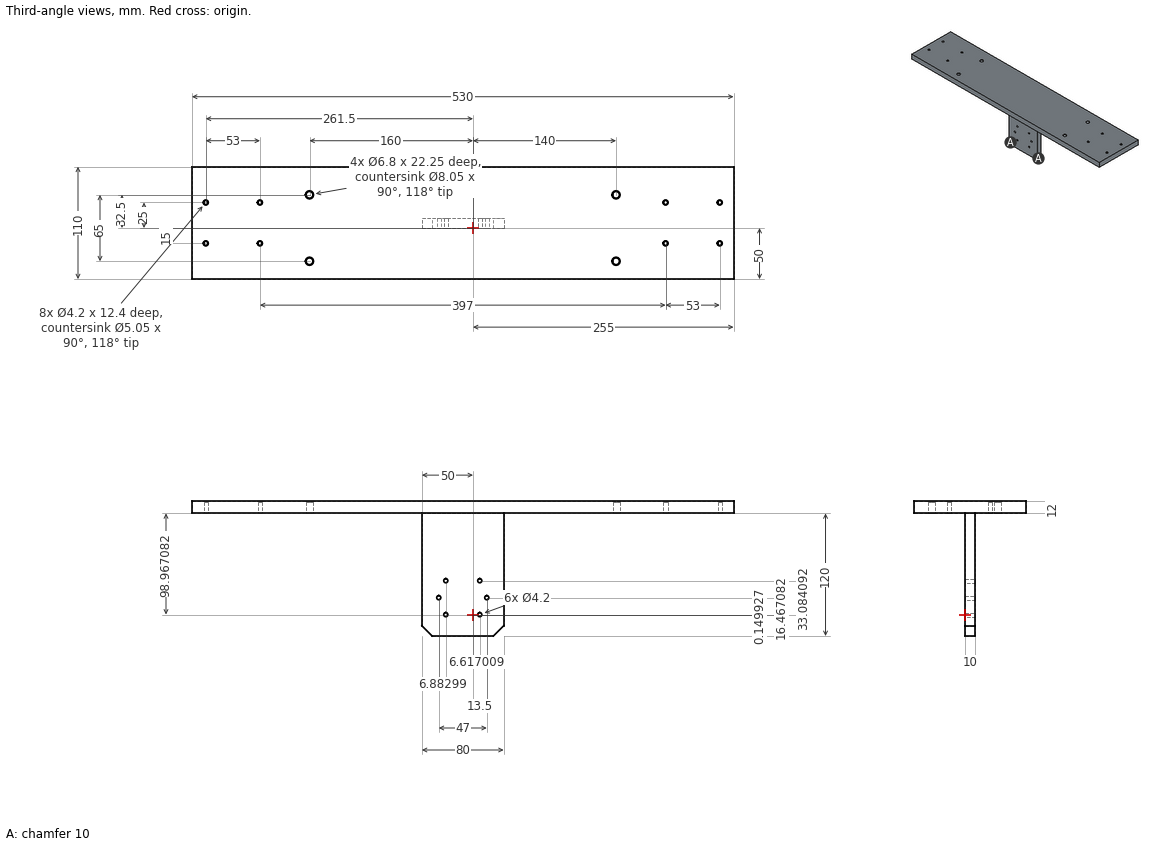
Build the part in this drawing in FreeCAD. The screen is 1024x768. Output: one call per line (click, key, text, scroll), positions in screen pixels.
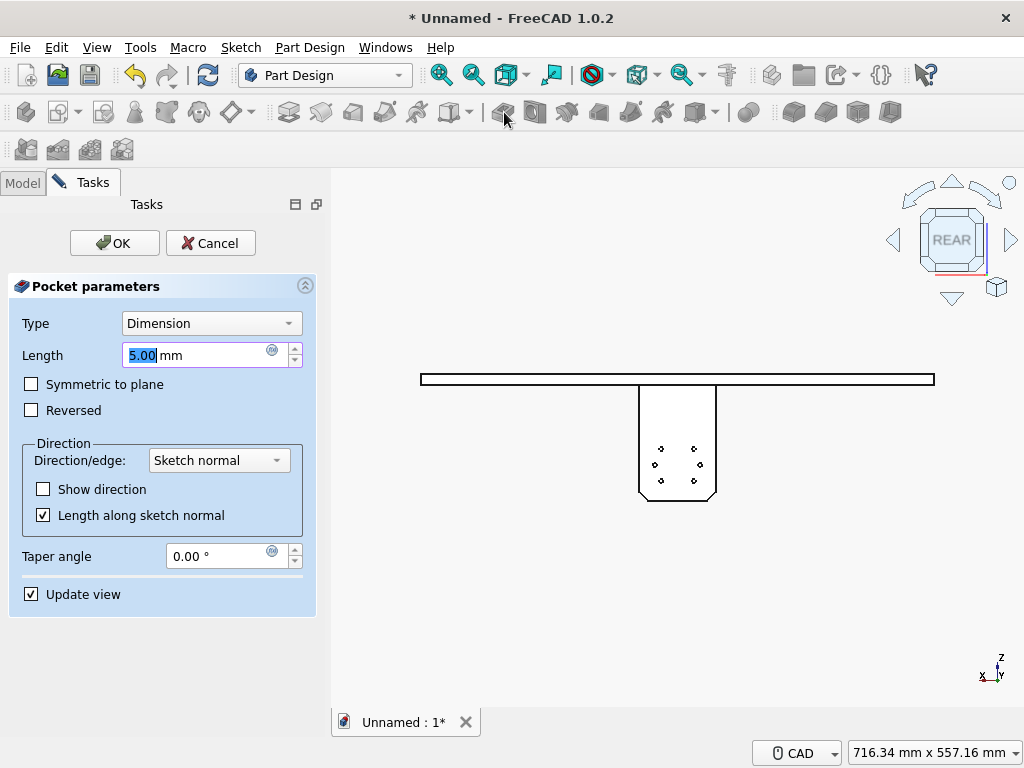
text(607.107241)
key(Tab)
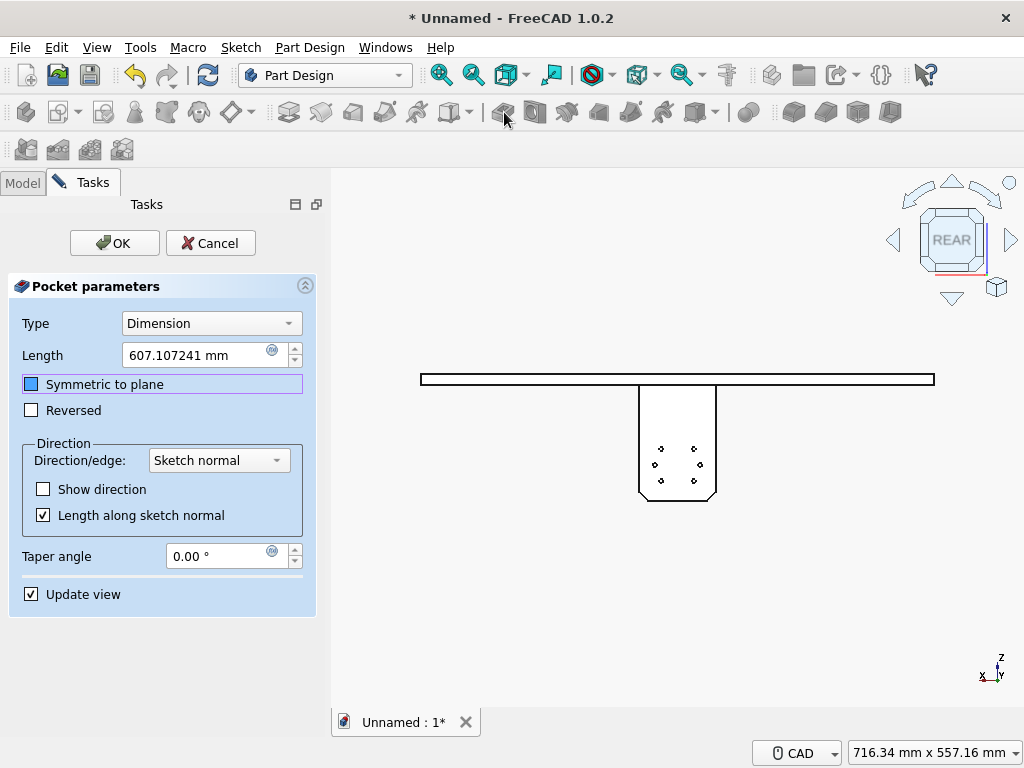
click(30, 384)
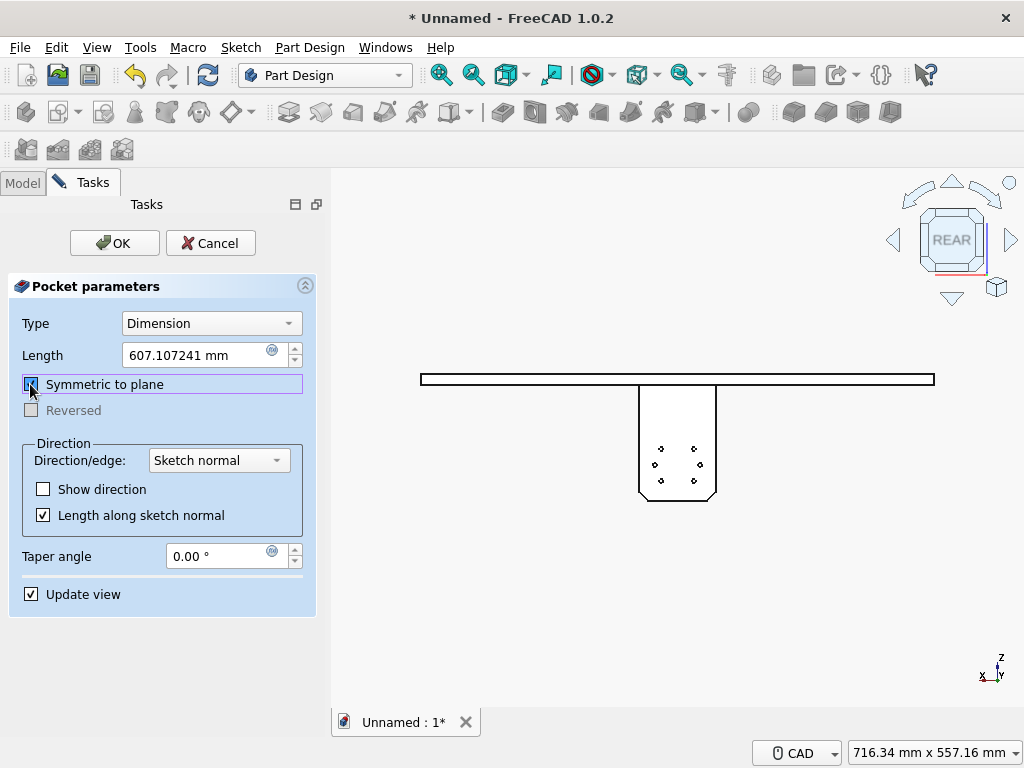
click(115, 243)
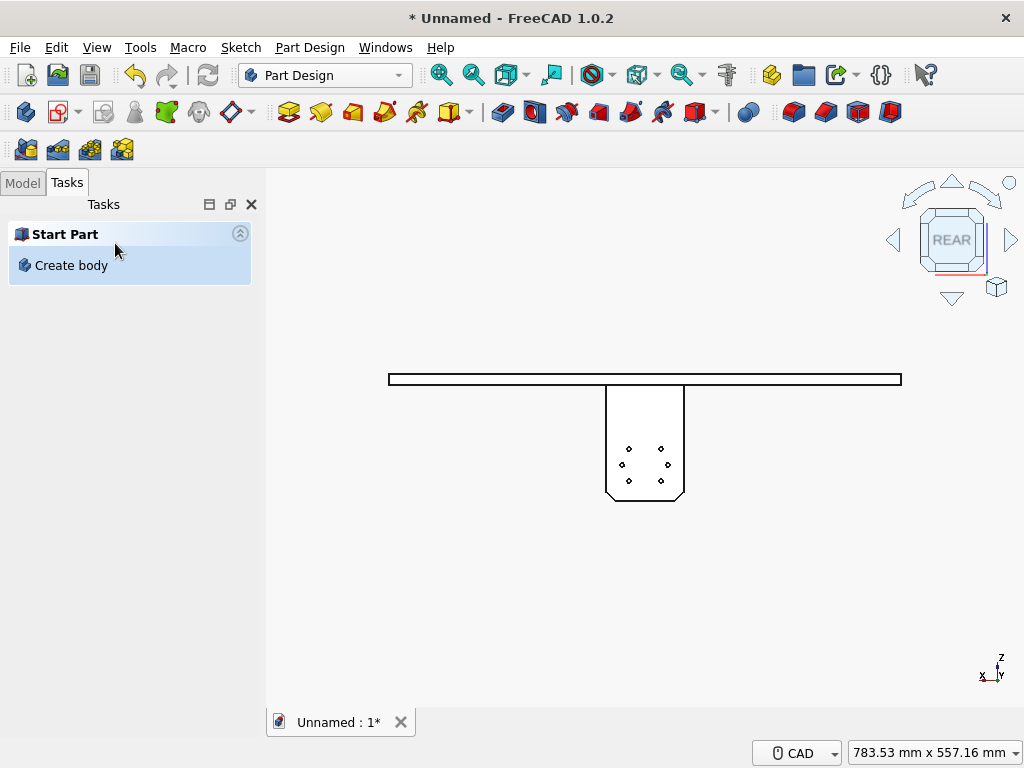
key(0)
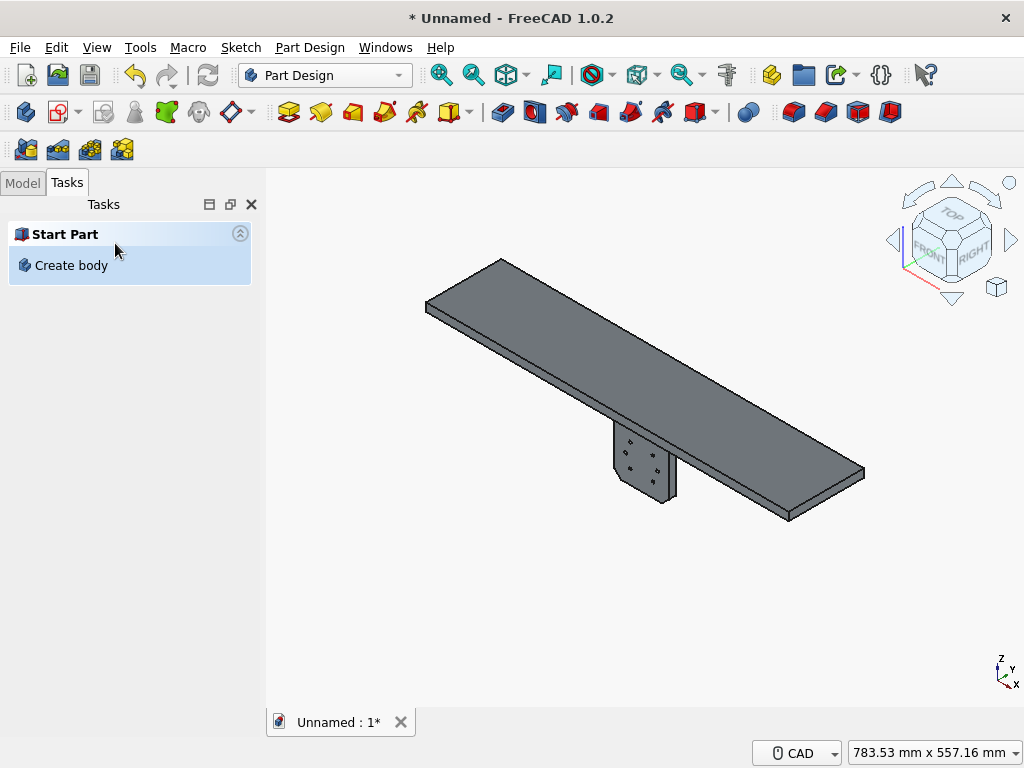
click(749, 444)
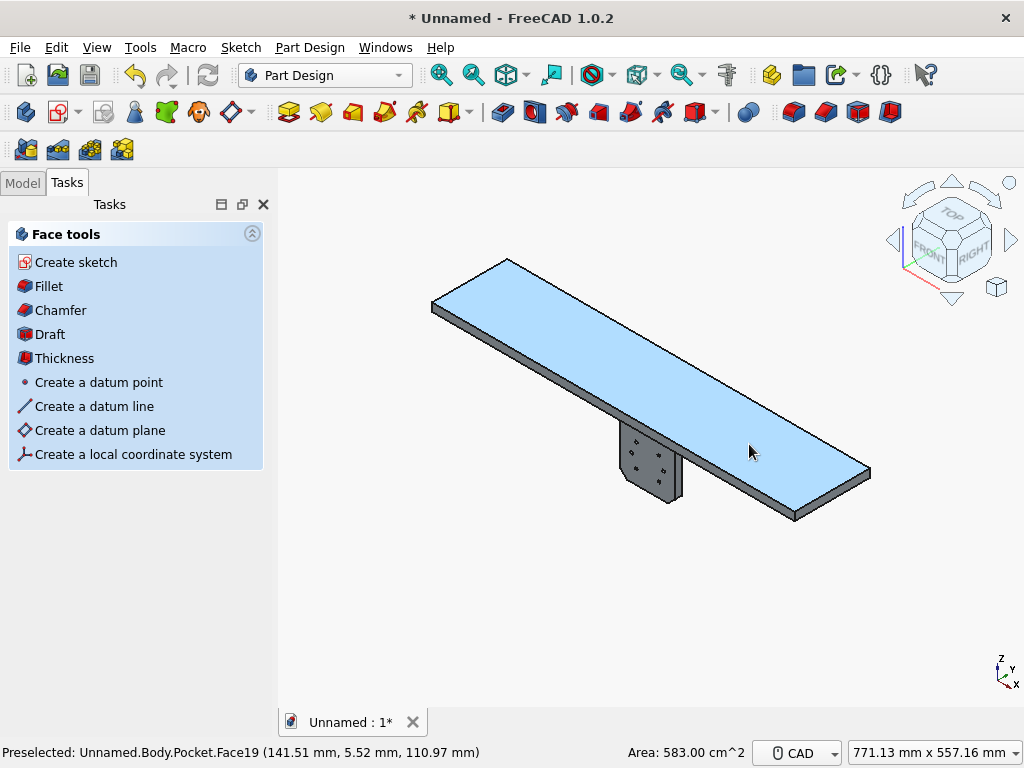
click(58, 112)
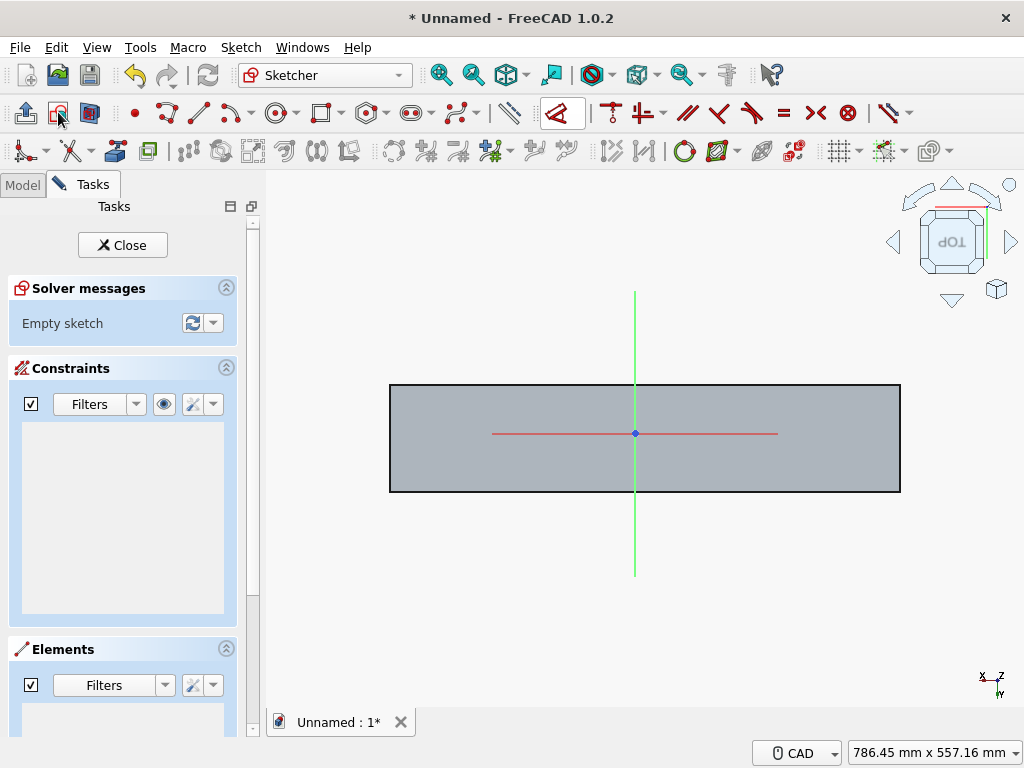
scroll(294, 439, down, 1)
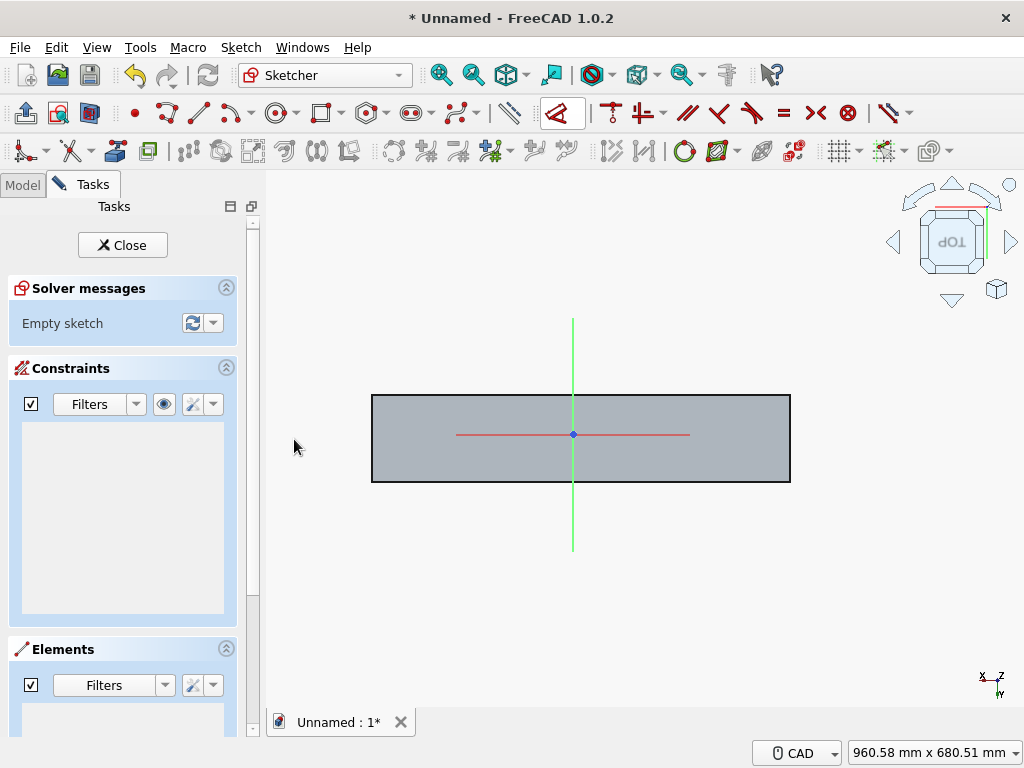
click(276, 114)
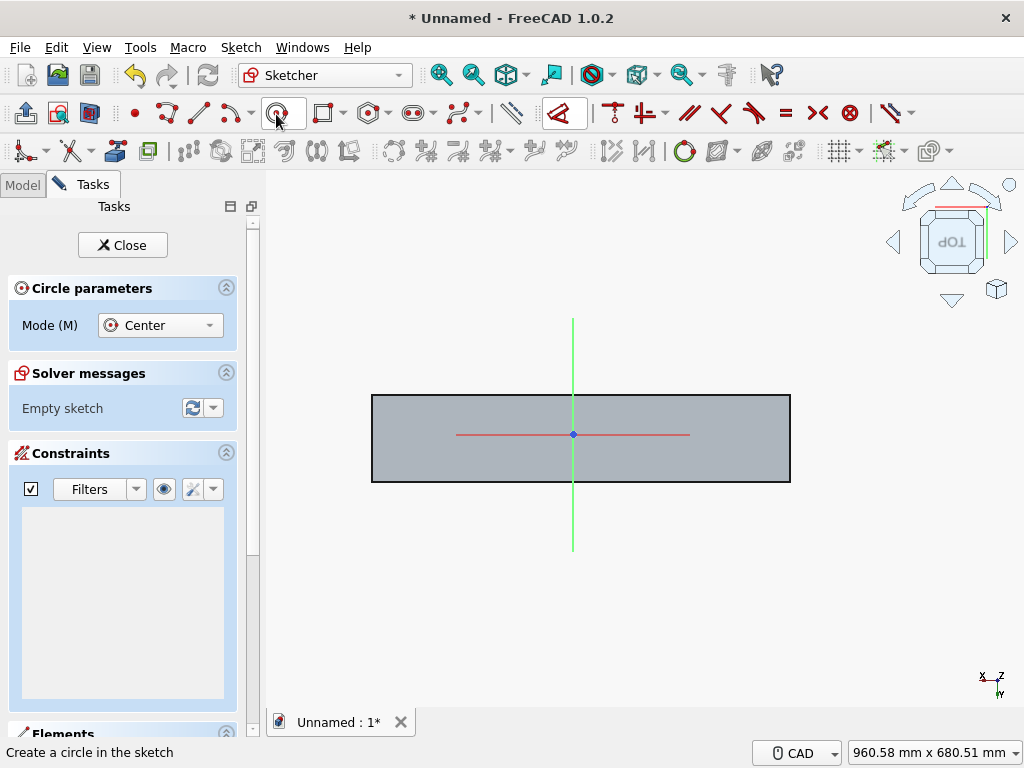
scroll(780, 454, up, 14)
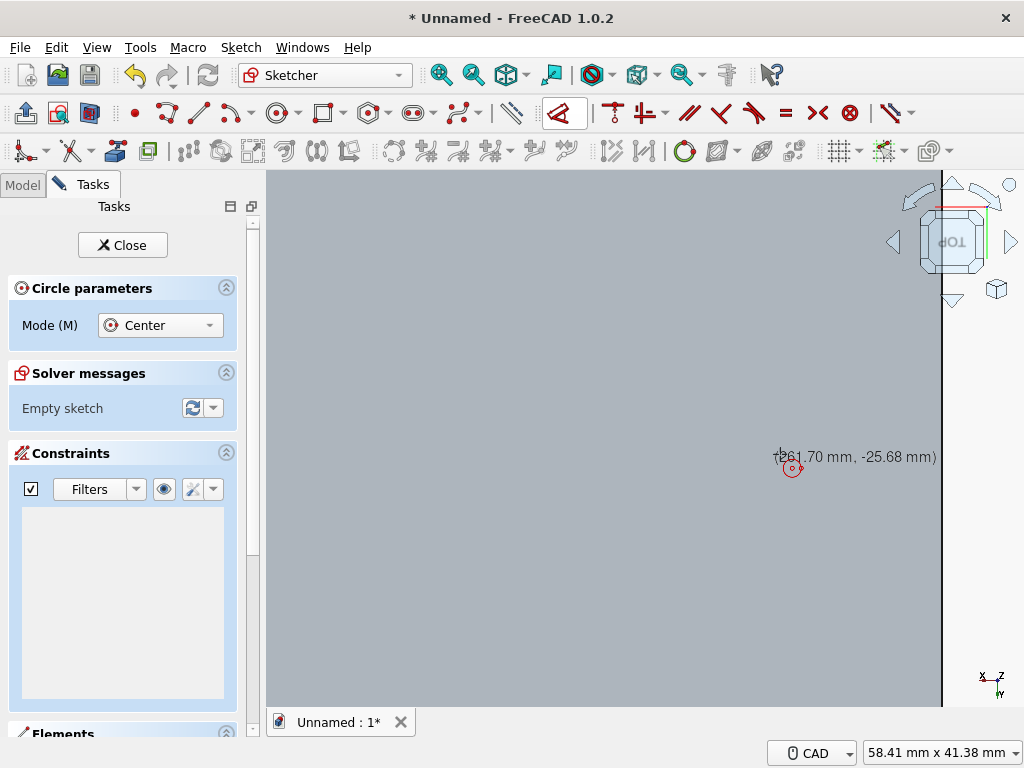
scroll(775, 454, down, 14)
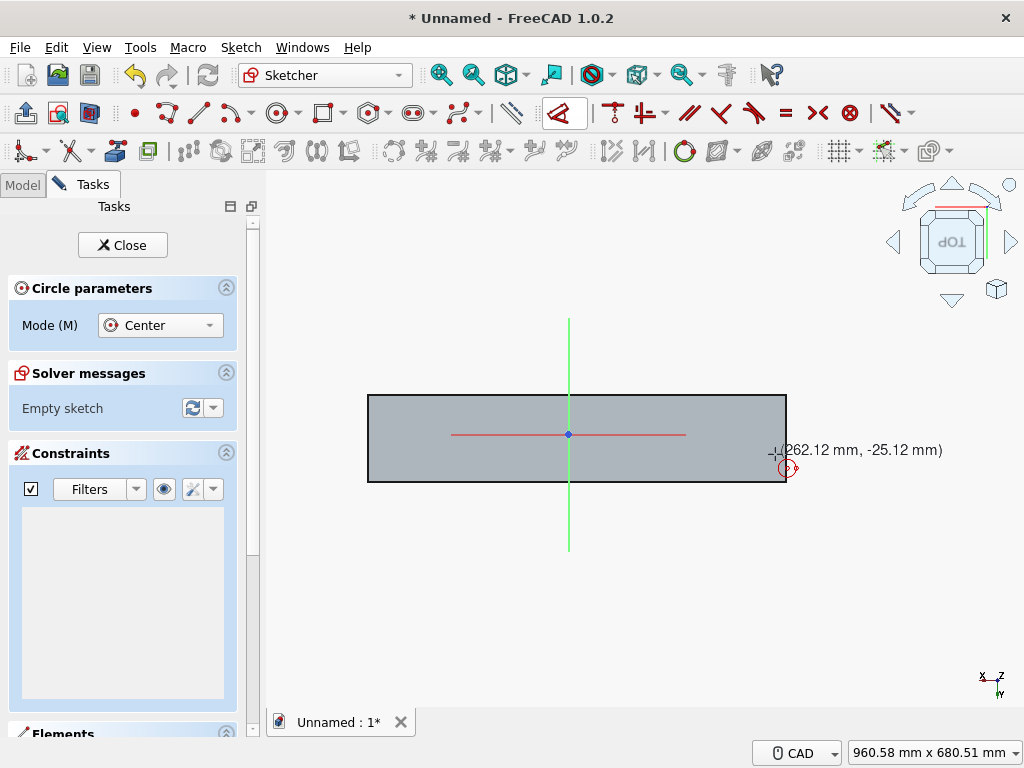
click(775, 454)
move(776, 453)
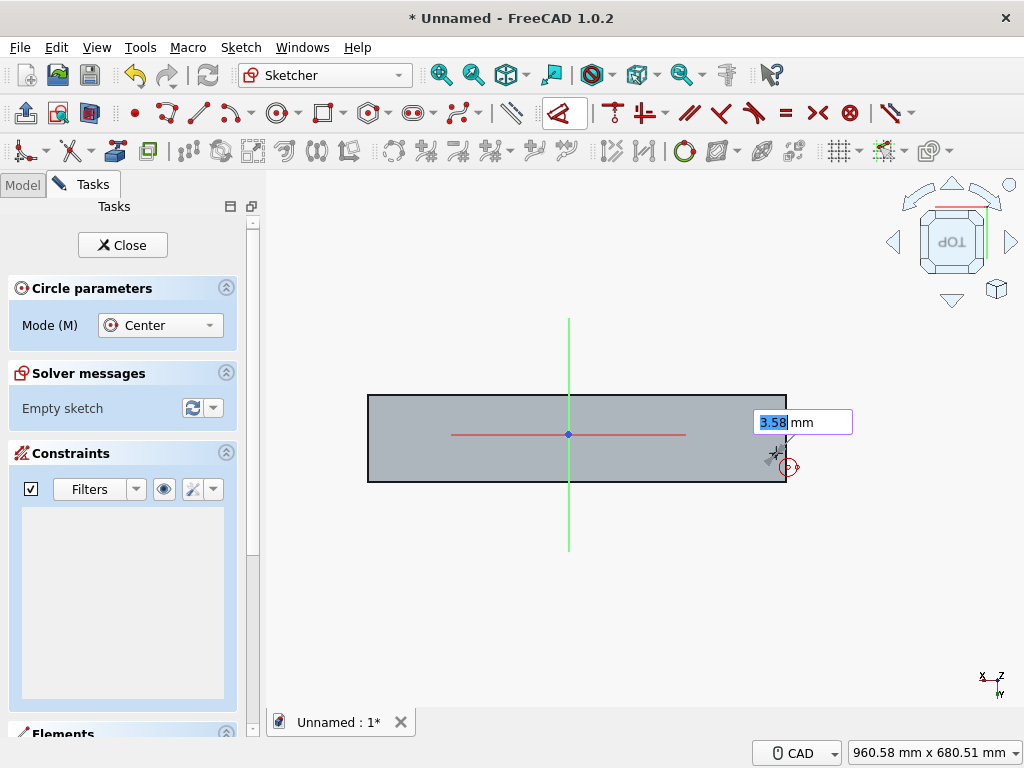
text(4.2)
key(Return)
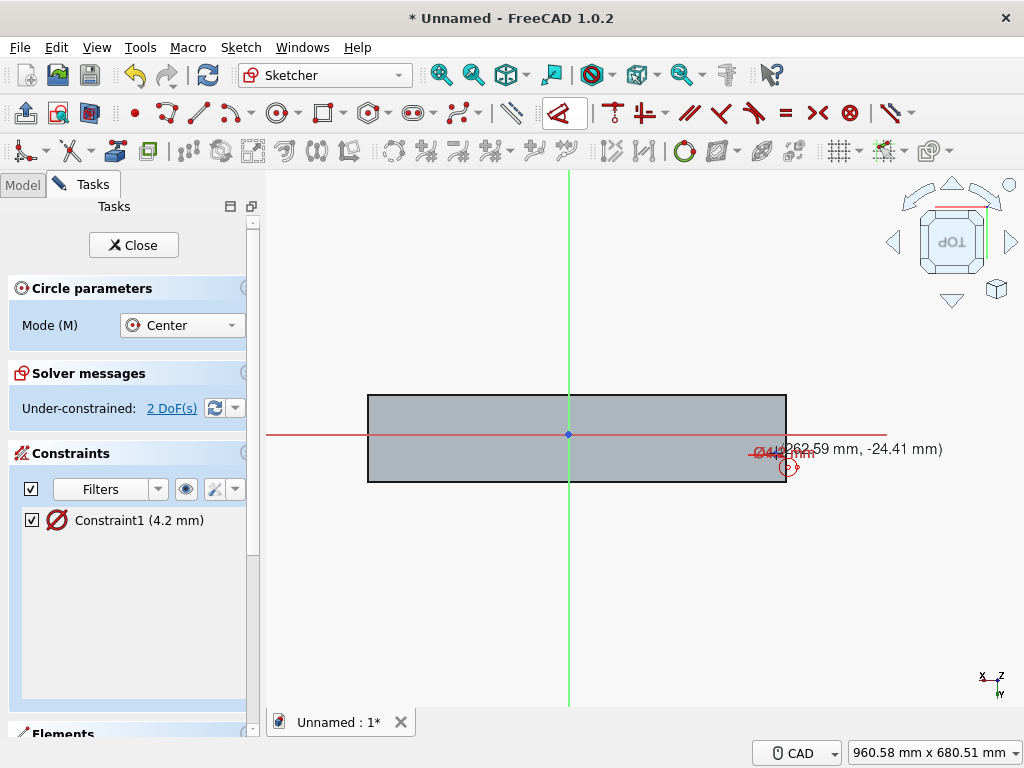
scroll(775, 423, up, 14)